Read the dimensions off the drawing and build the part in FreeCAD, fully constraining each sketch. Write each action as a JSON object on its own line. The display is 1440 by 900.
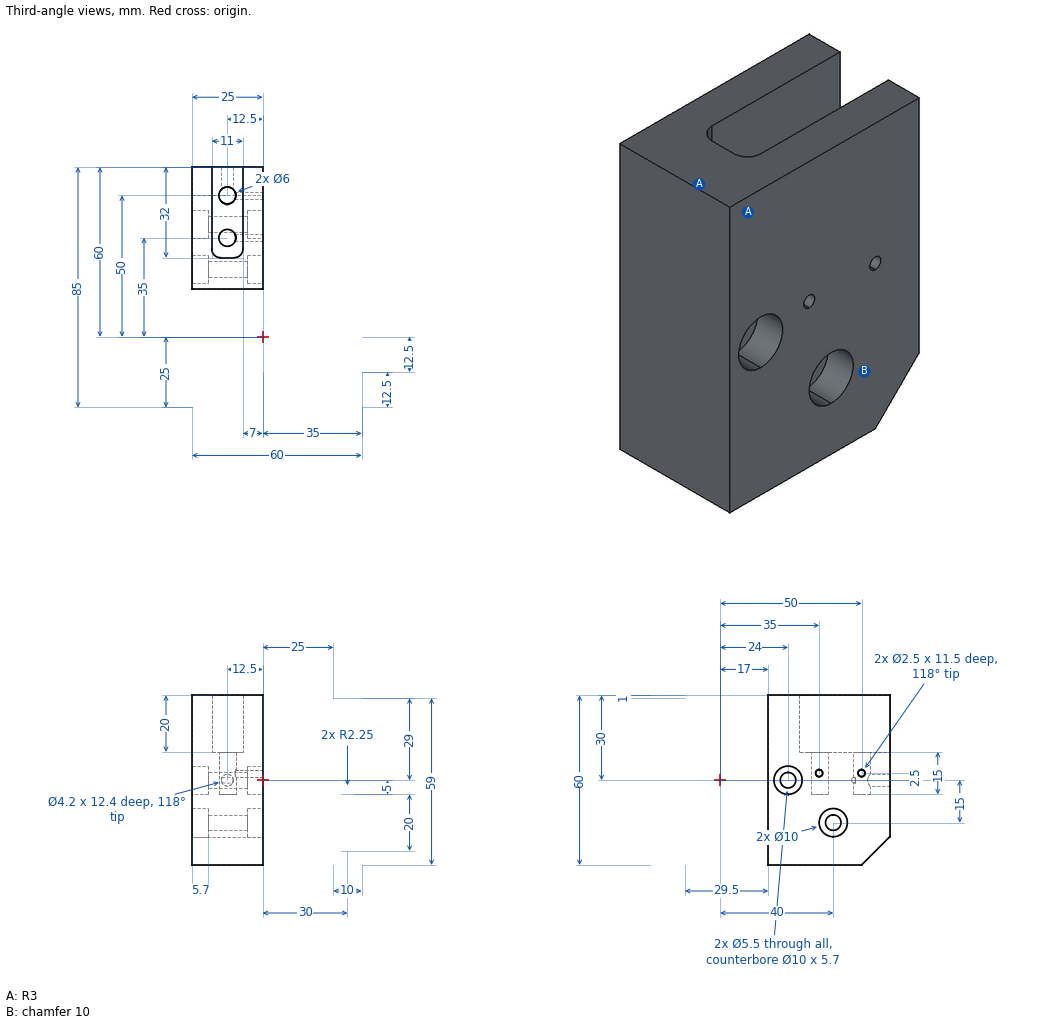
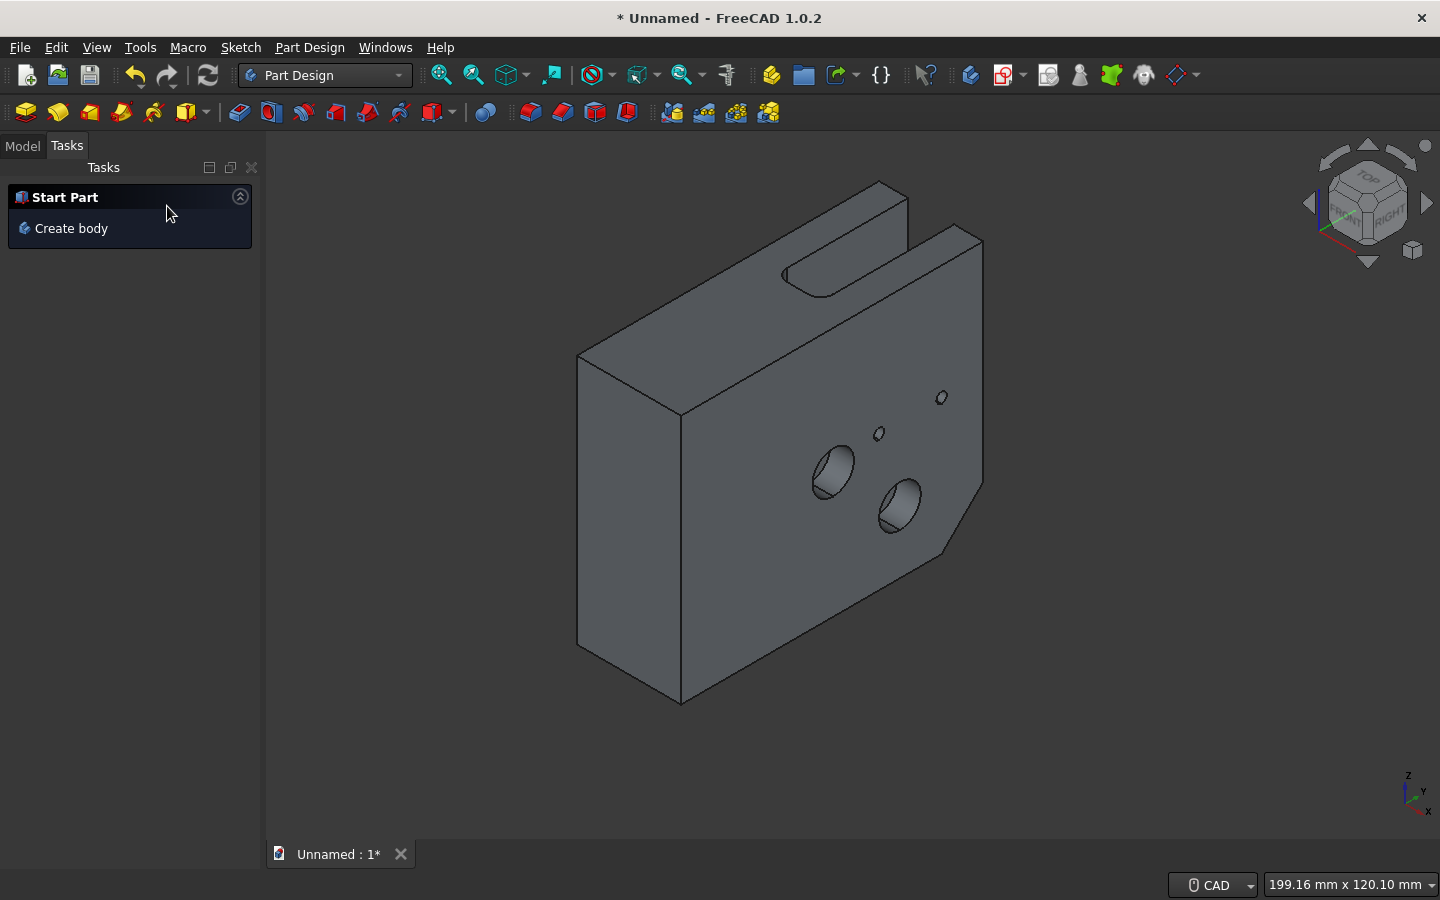
{"action": "key", "text": "6"}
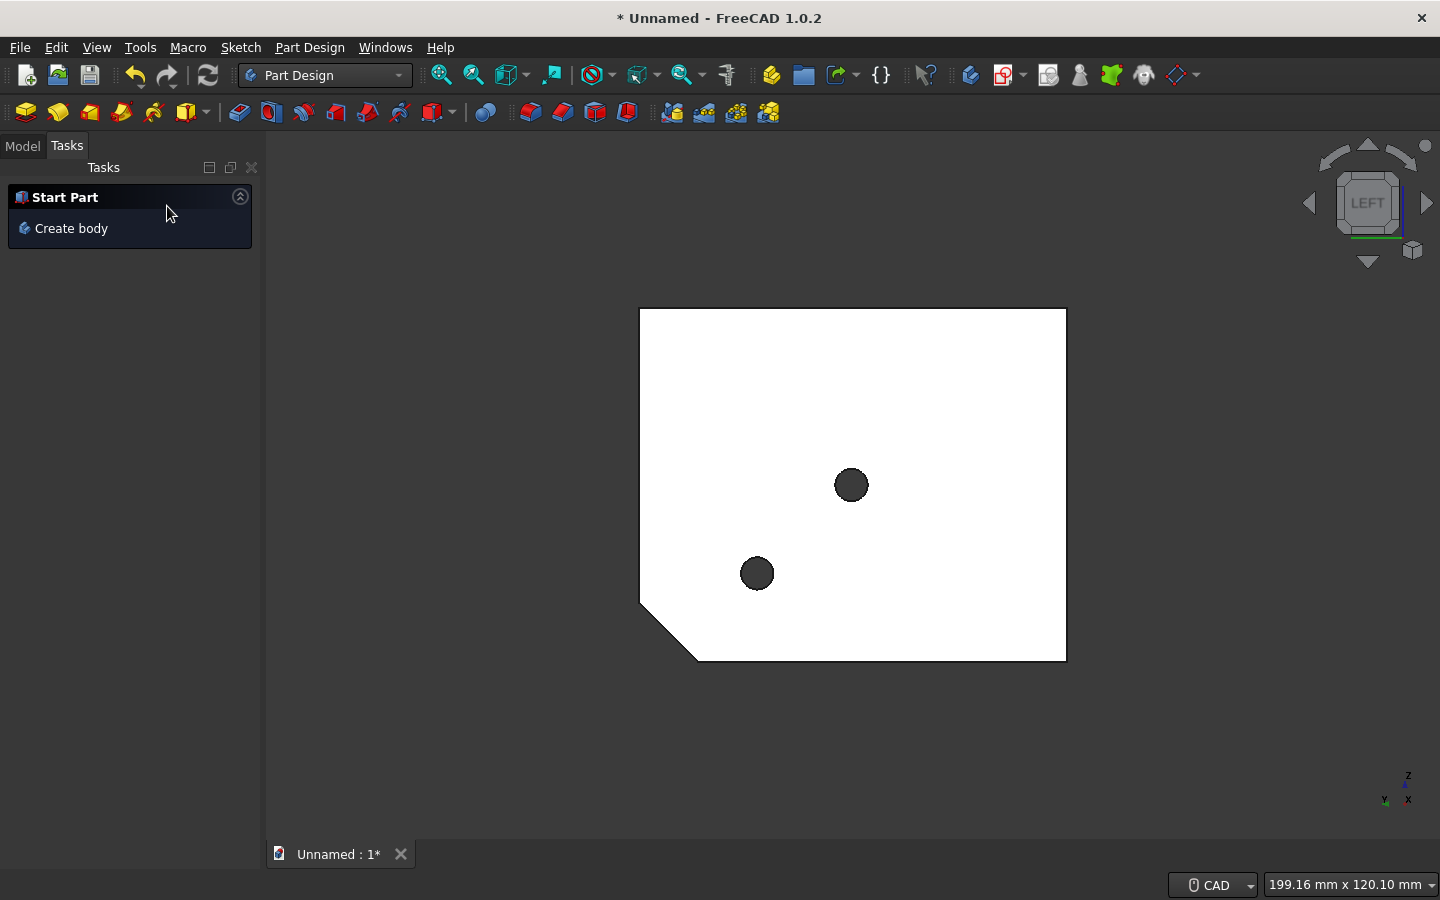
{"action": "left_click", "coordinate": [731, 433]}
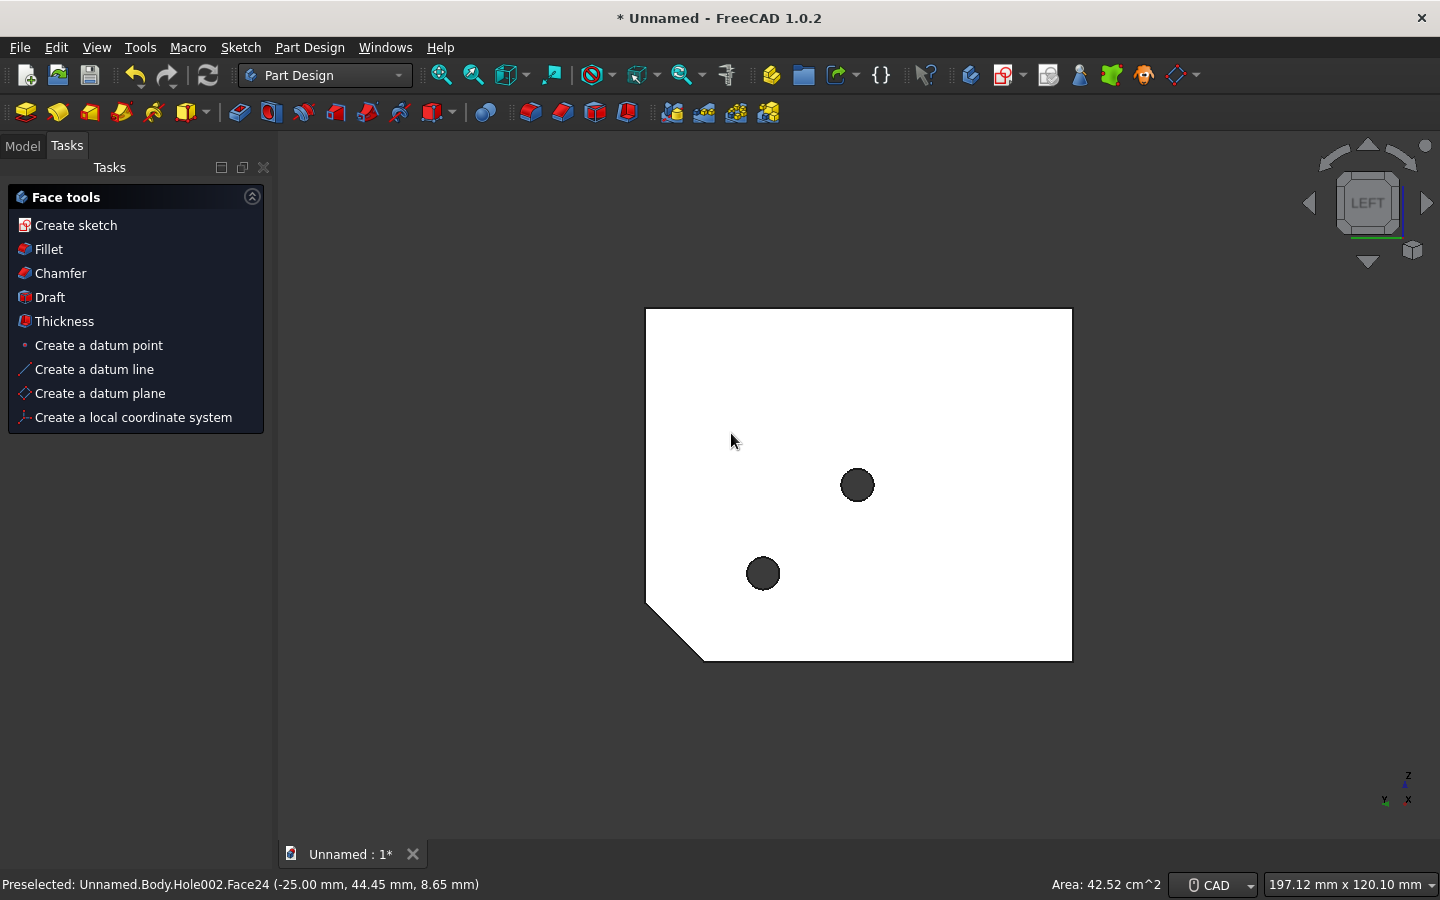
{"action": "left_click", "coordinate": [1004, 76]}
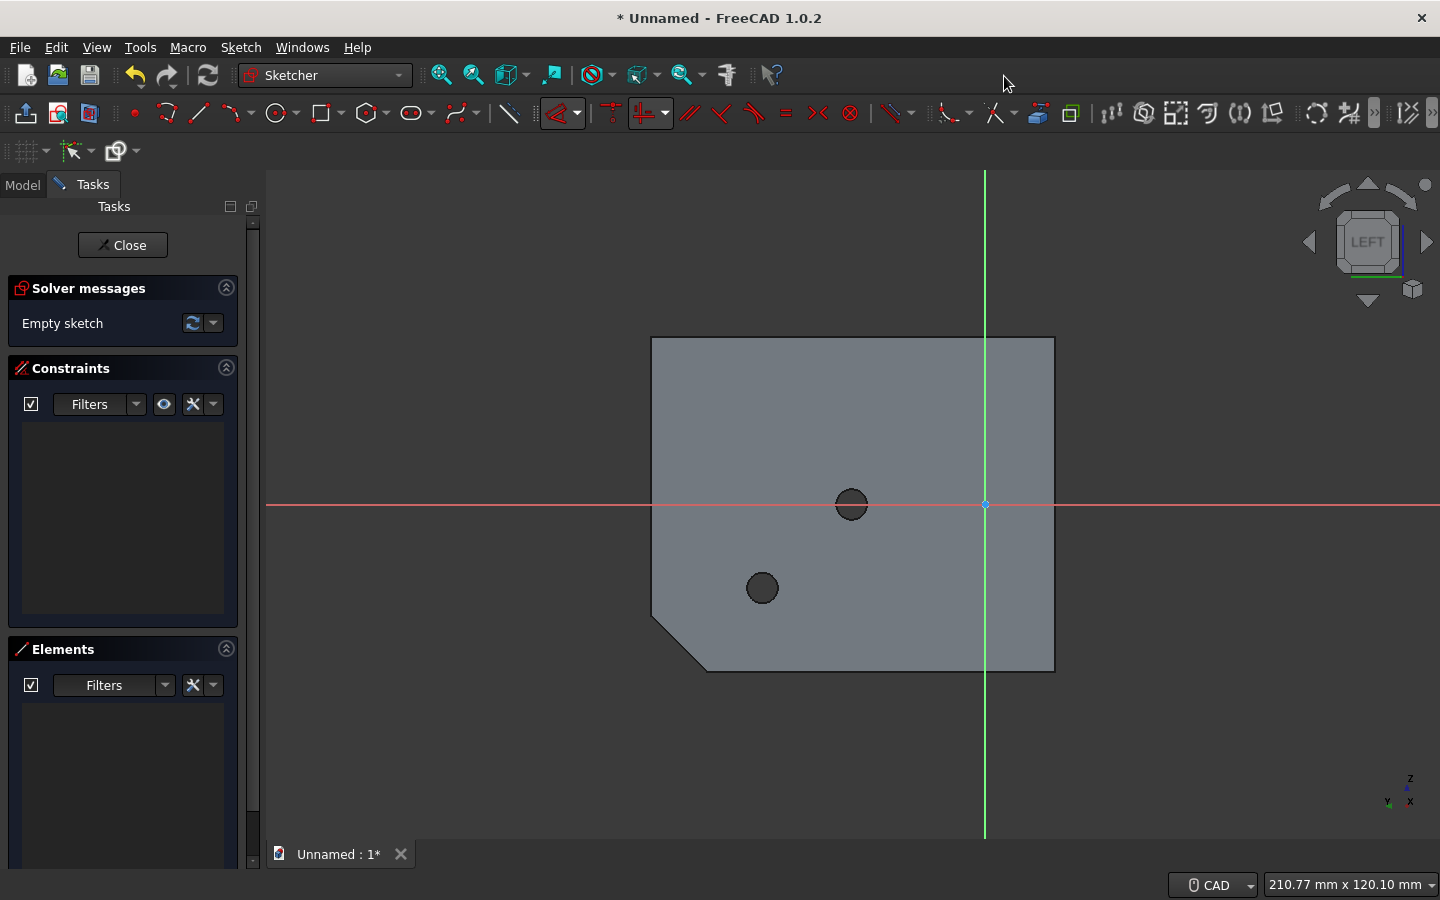
{"action": "left_click", "coordinate": [322, 114]}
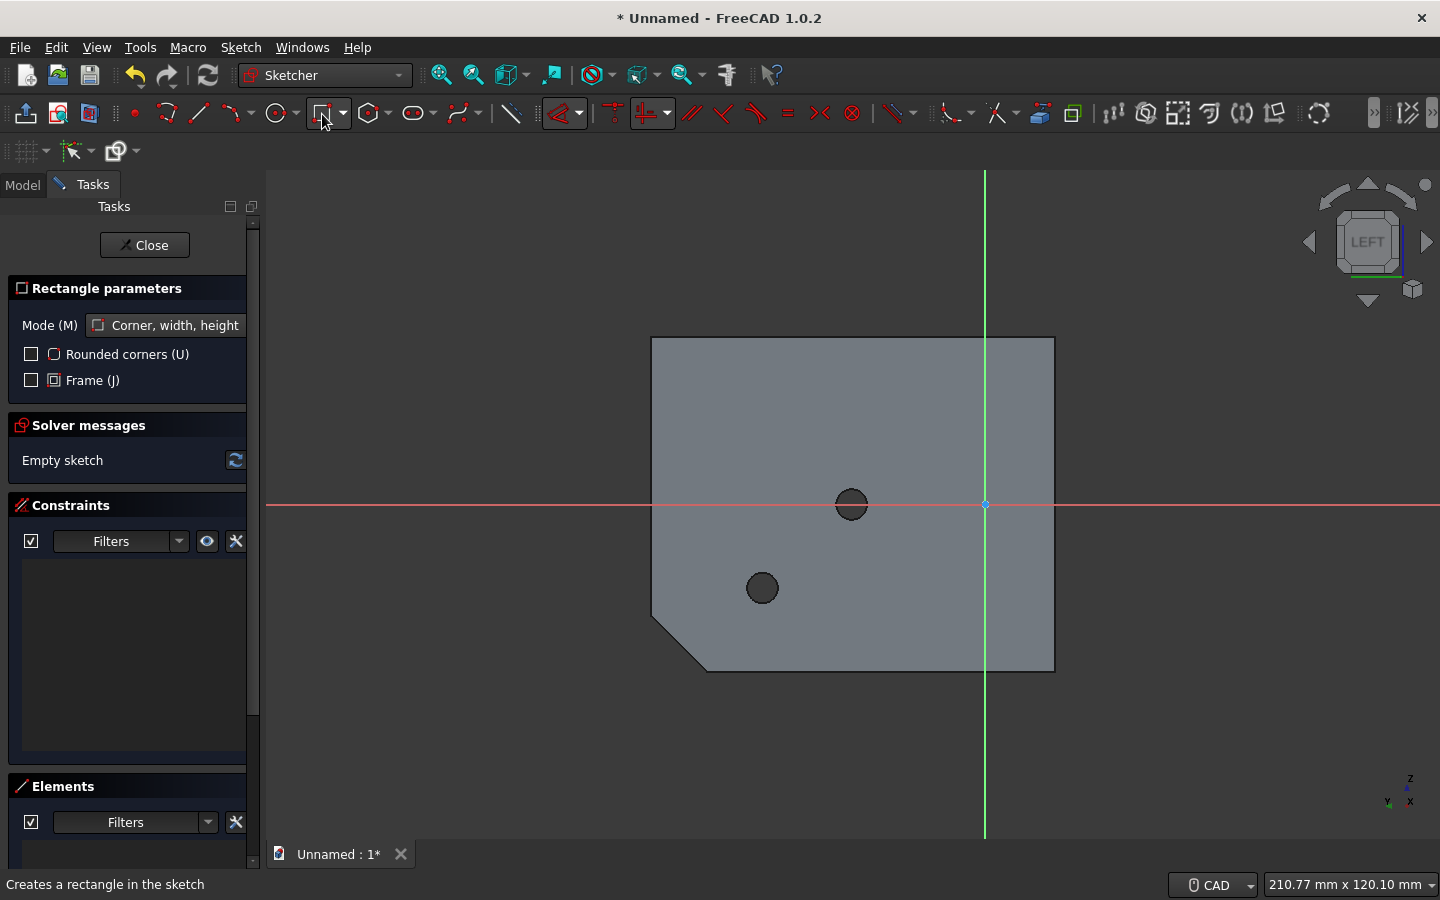
{"action": "left_click", "coordinate": [891, 337]}
{"action": "mouse_move", "coordinate": [1055, 672]}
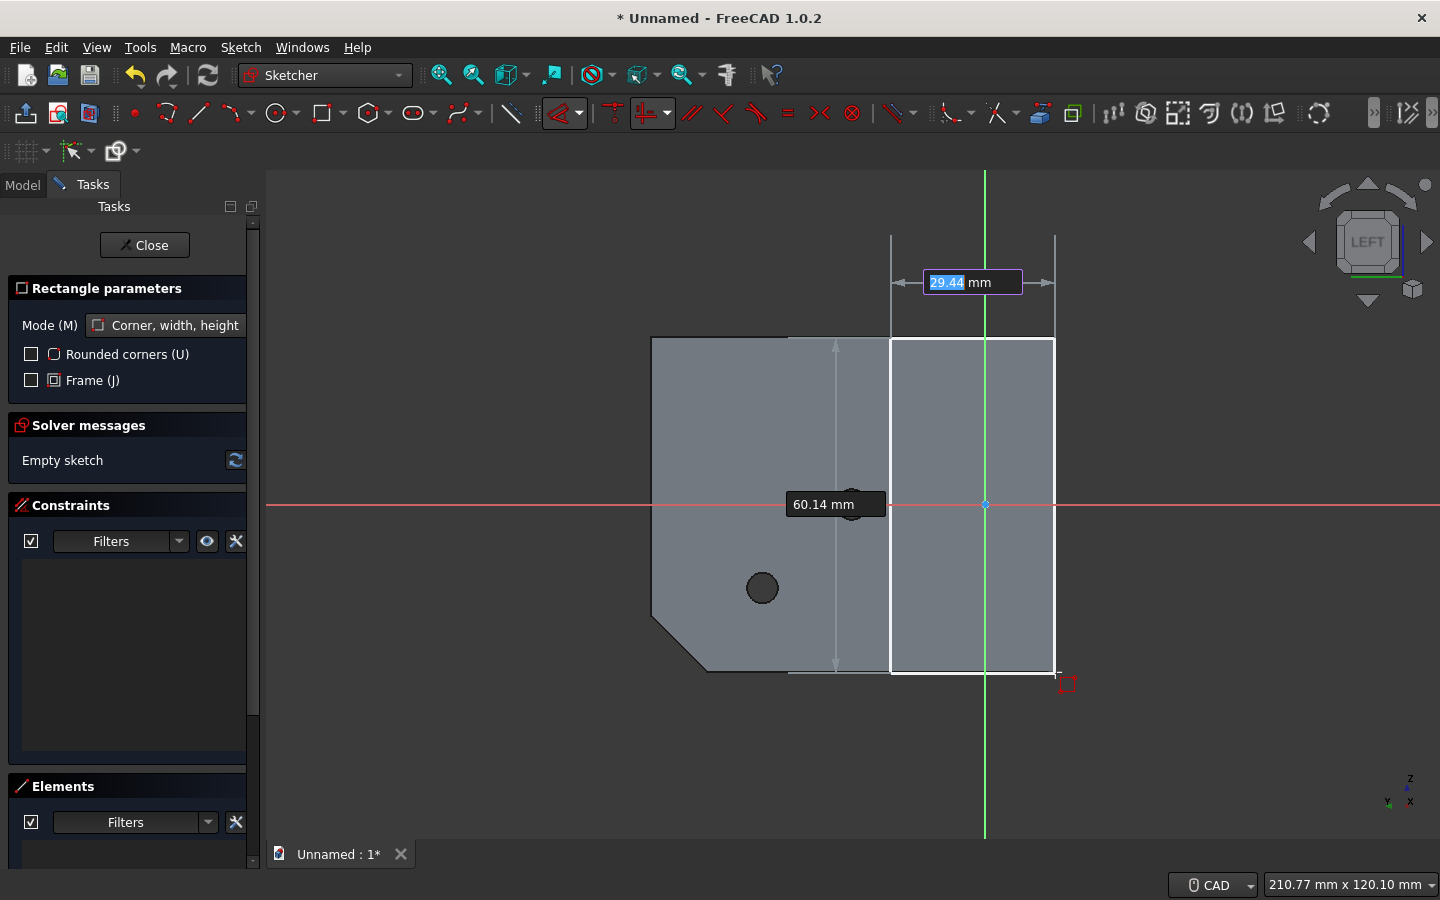
{"action": "type", "text": "29.5"}
{"action": "key", "text": "Tab"}
{"action": "type", "text": "60"}
{"action": "key", "text": "Return"}
{"action": "key", "text": "Escape"}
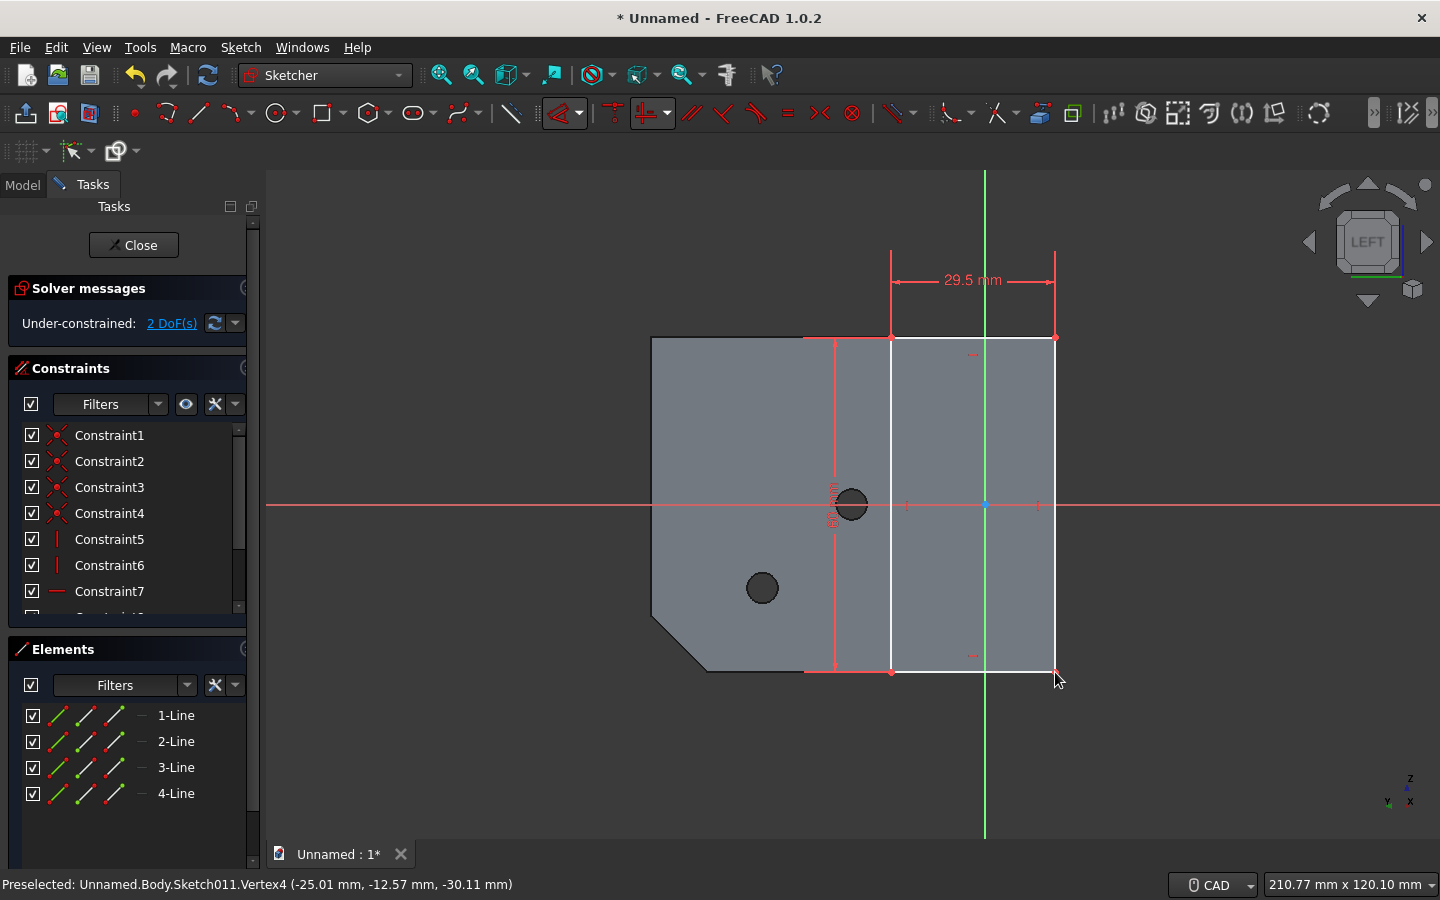
{"action": "left_click", "coordinate": [891, 338]}